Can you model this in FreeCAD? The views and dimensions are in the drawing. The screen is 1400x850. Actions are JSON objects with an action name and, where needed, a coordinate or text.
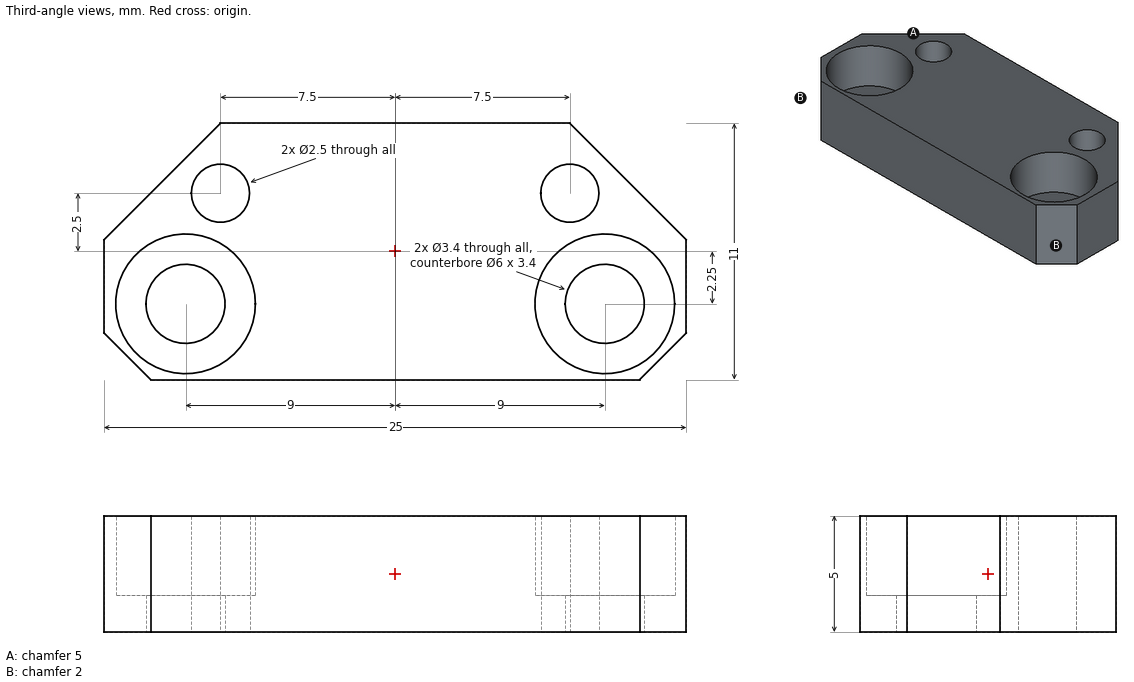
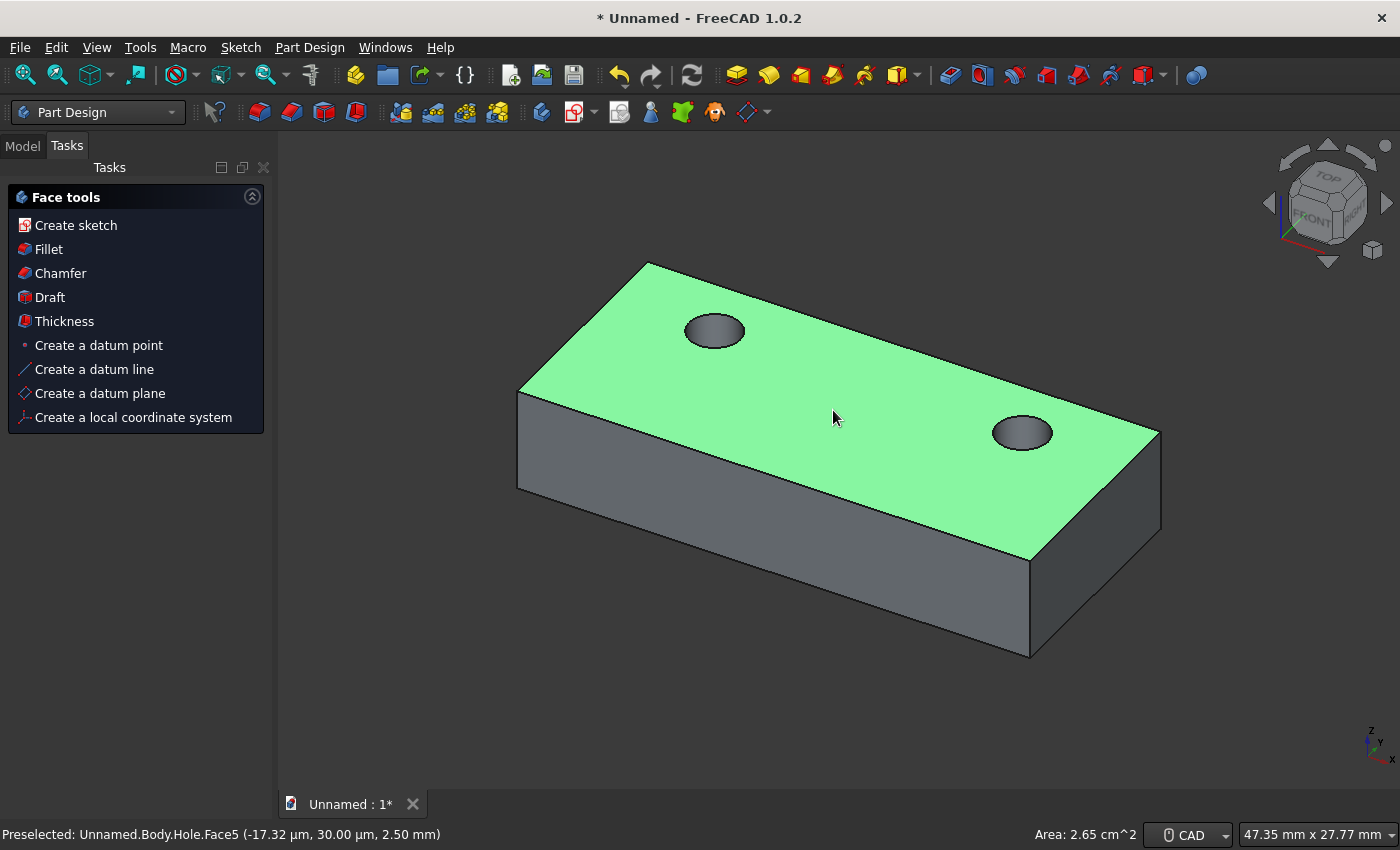
{"action": "left_click", "coordinate": [574, 112]}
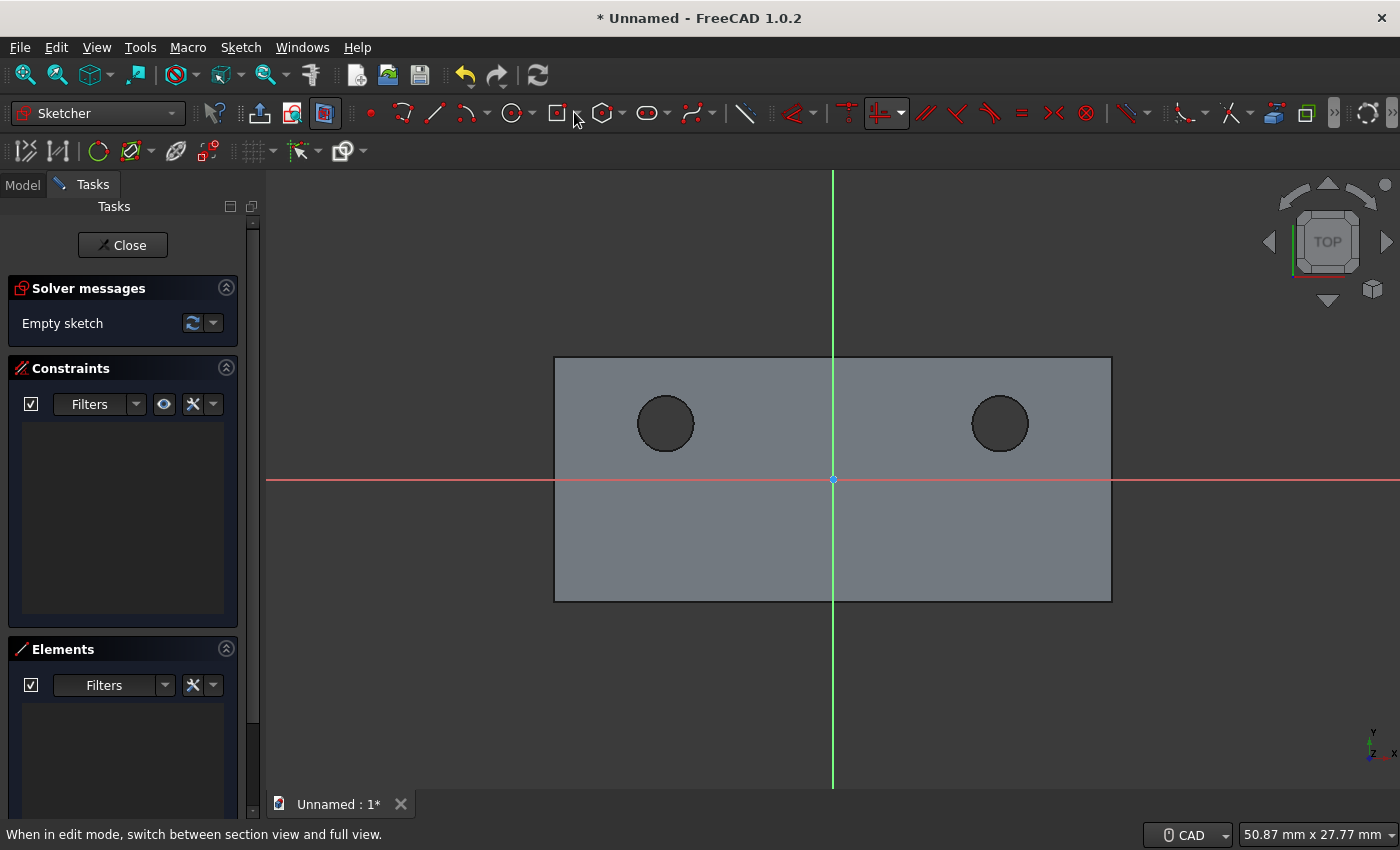
{"action": "scroll", "coordinate": [972, 613], "scroll_direction": "up", "scroll_amount": 2}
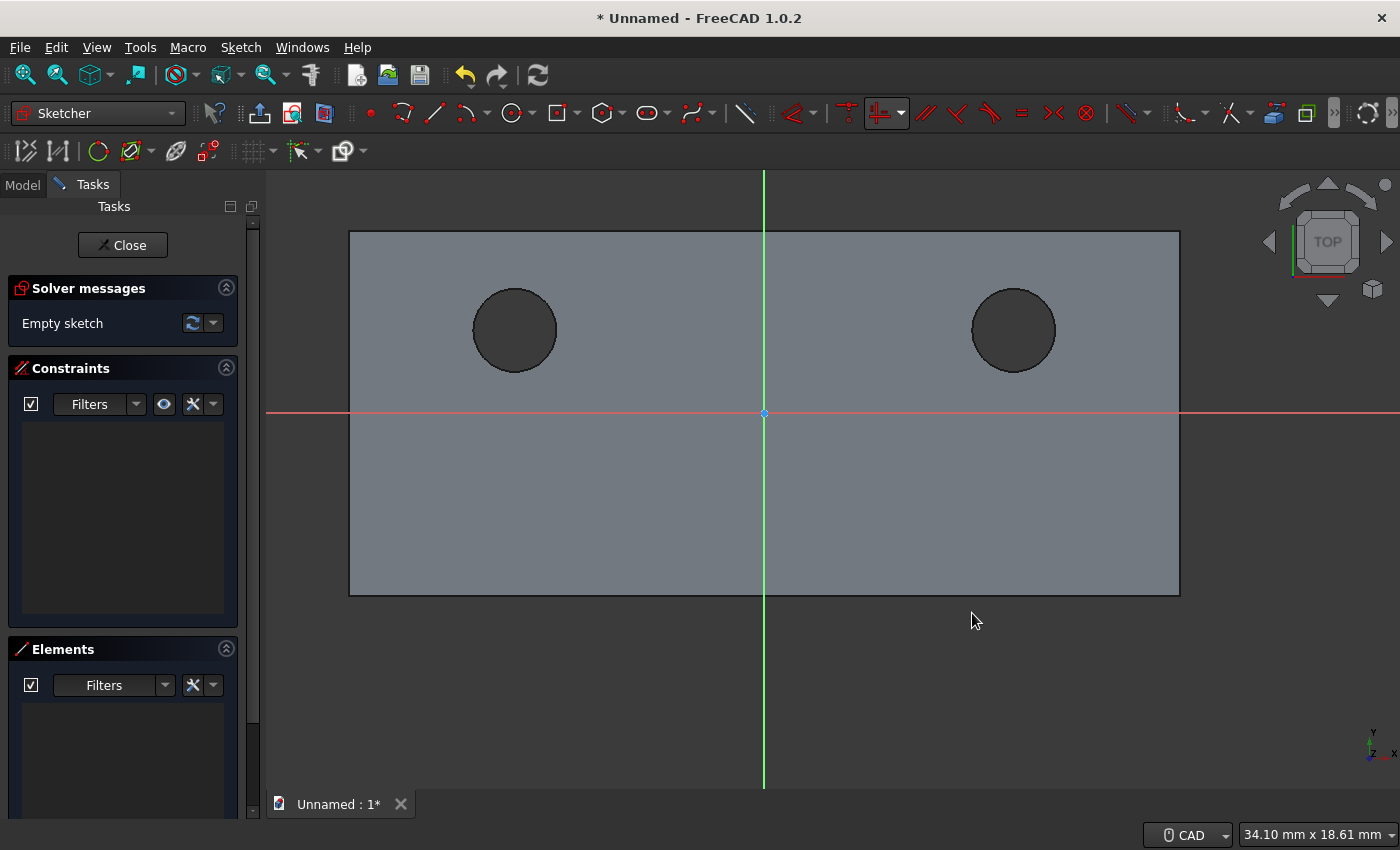
{"action": "left_click", "coordinate": [512, 114]}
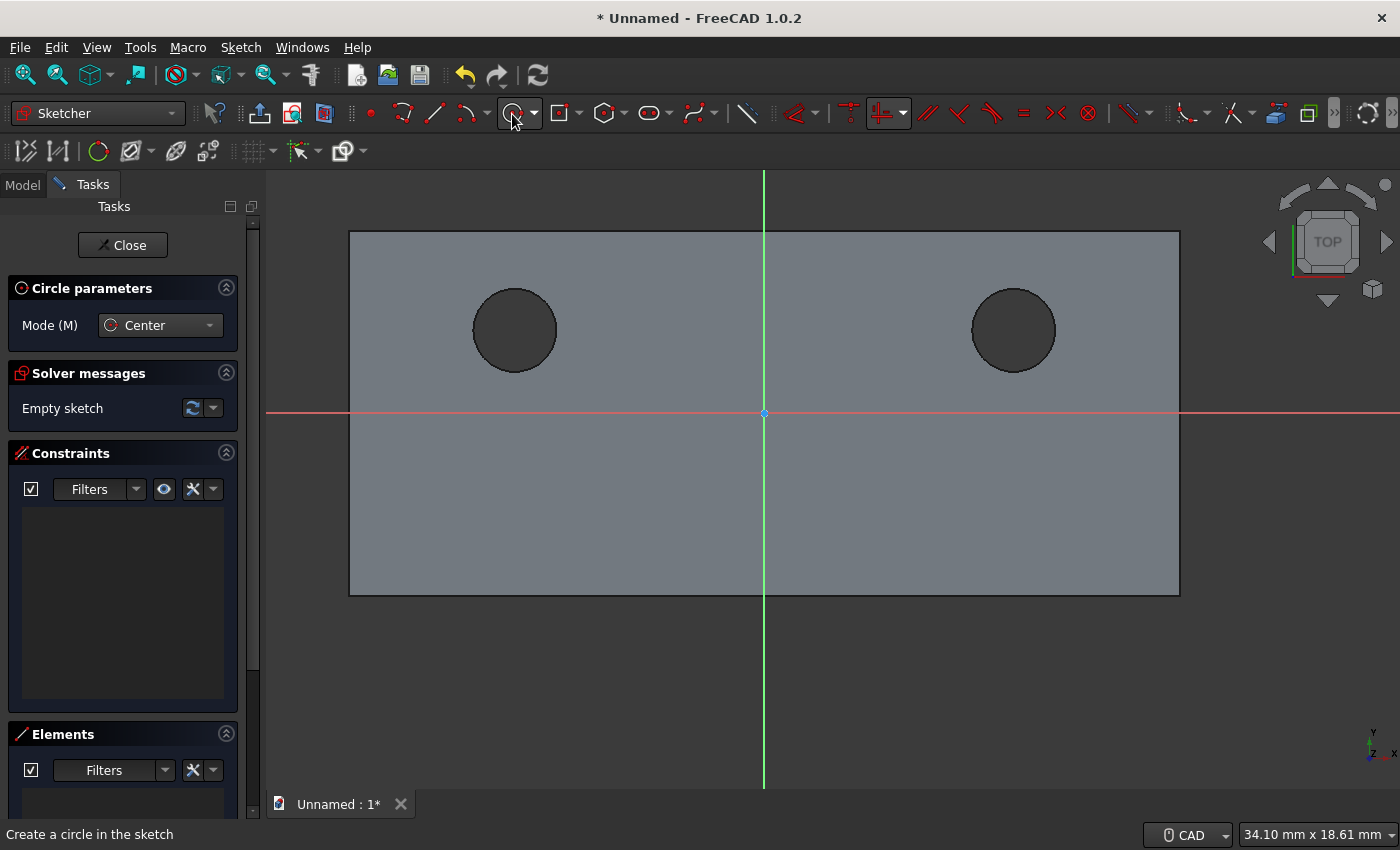
{"action": "left_click", "coordinate": [1064, 488]}
{"action": "left_click", "coordinate": [1104, 448]}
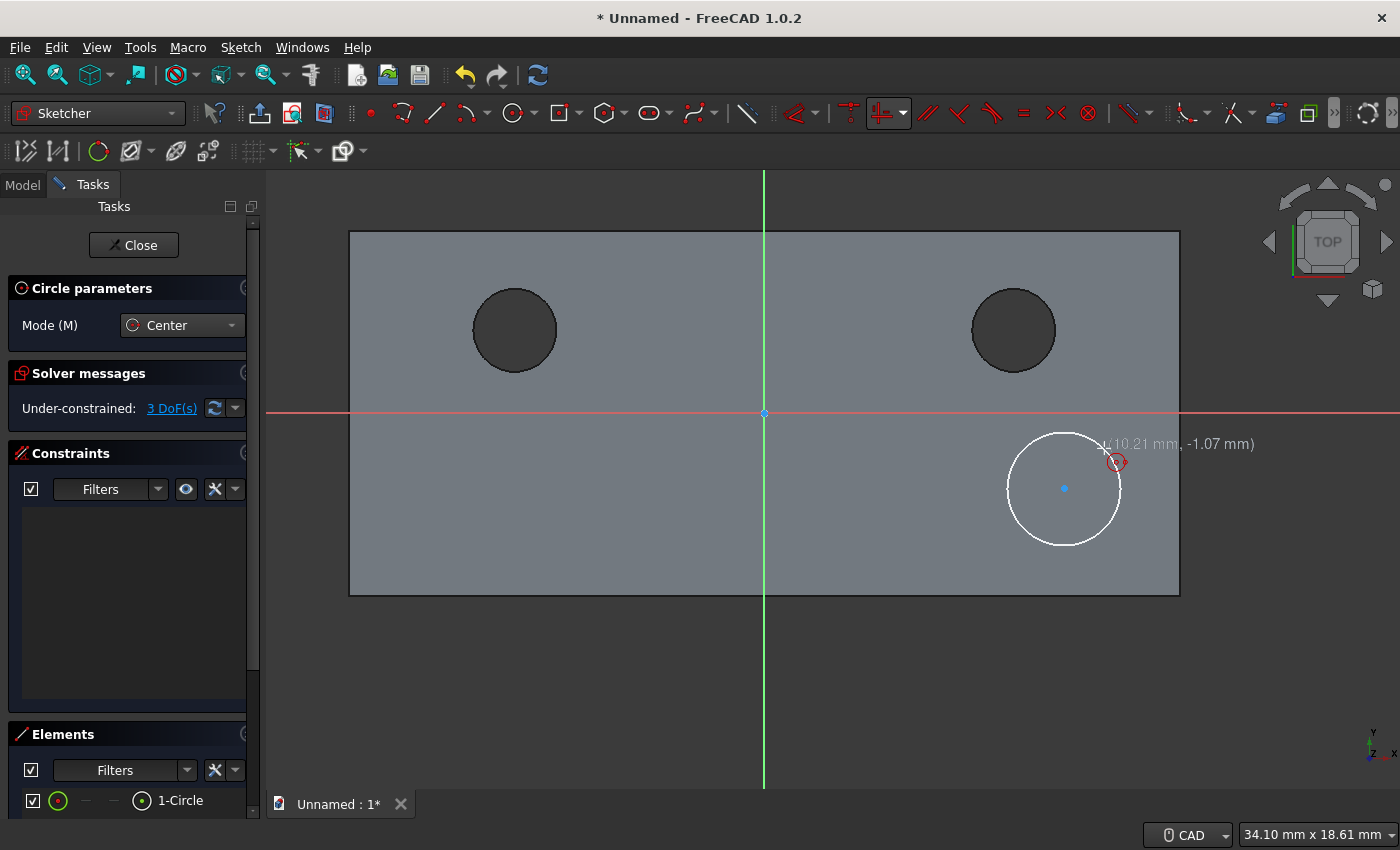
{"action": "left_click", "coordinate": [465, 488]}
{"action": "left_click", "coordinate": [505, 448]}
{"action": "key", "text": "Escape"}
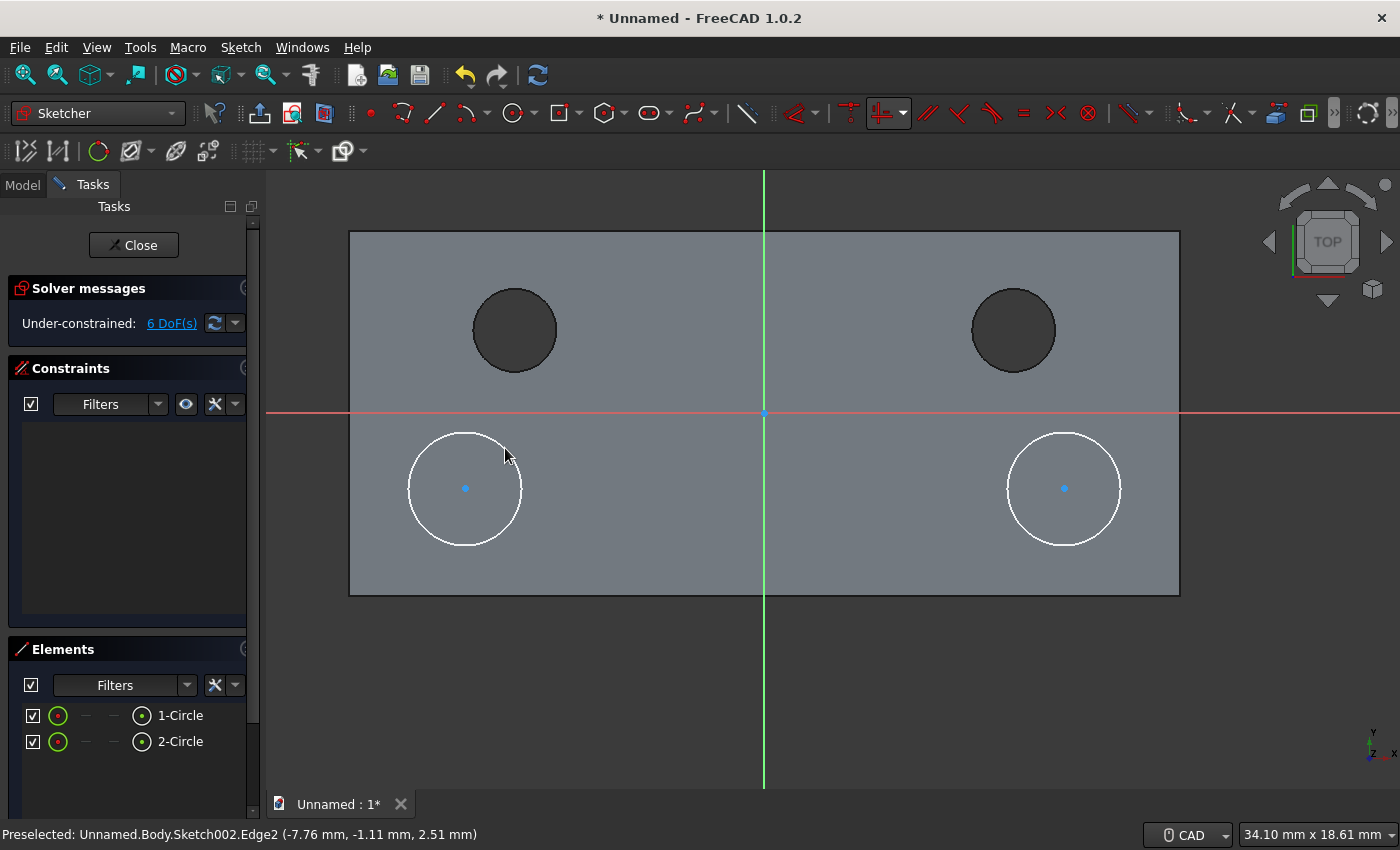
{"action": "left_click", "coordinate": [1104, 449]}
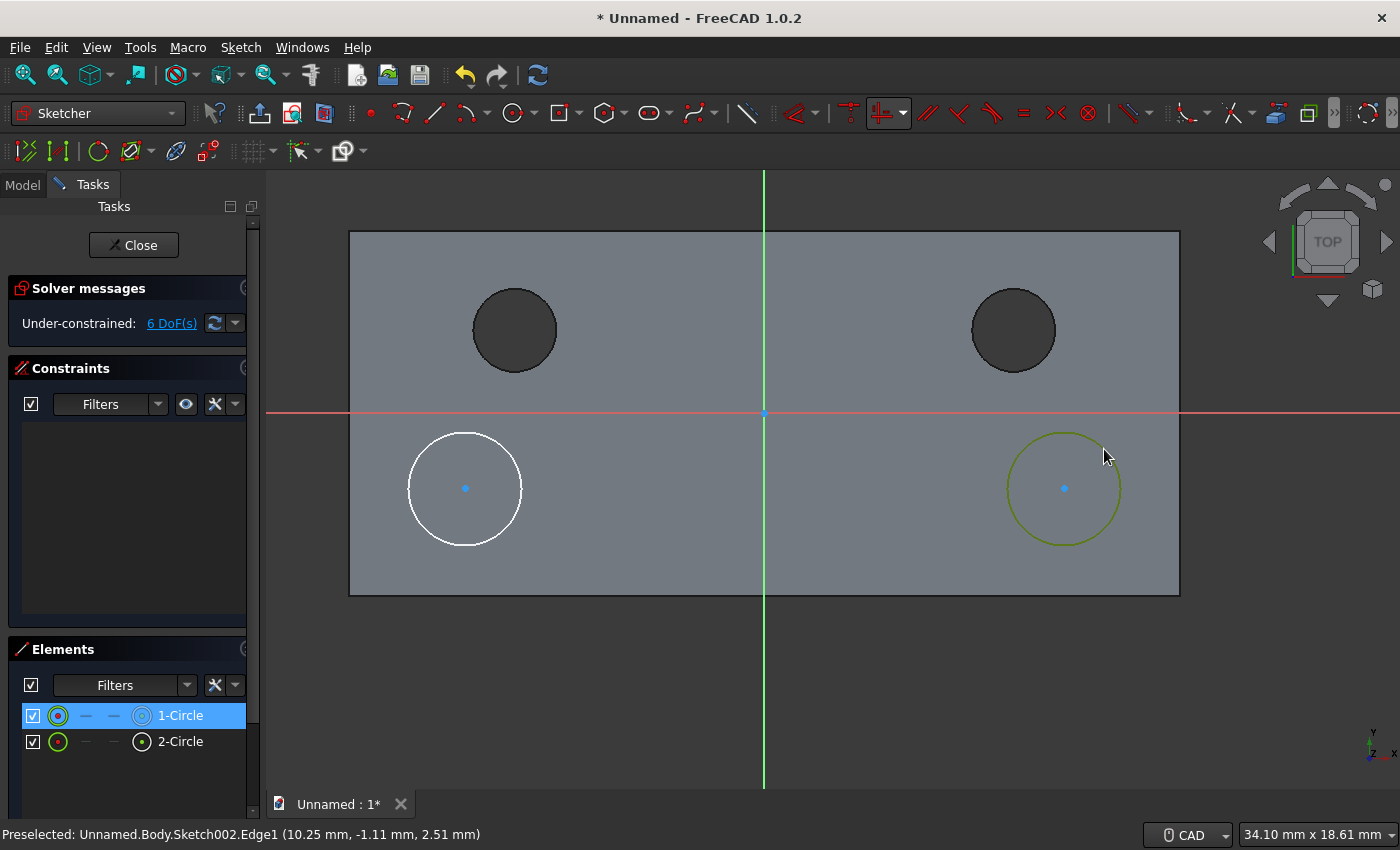
{"action": "left_click", "coordinate": [505, 449]}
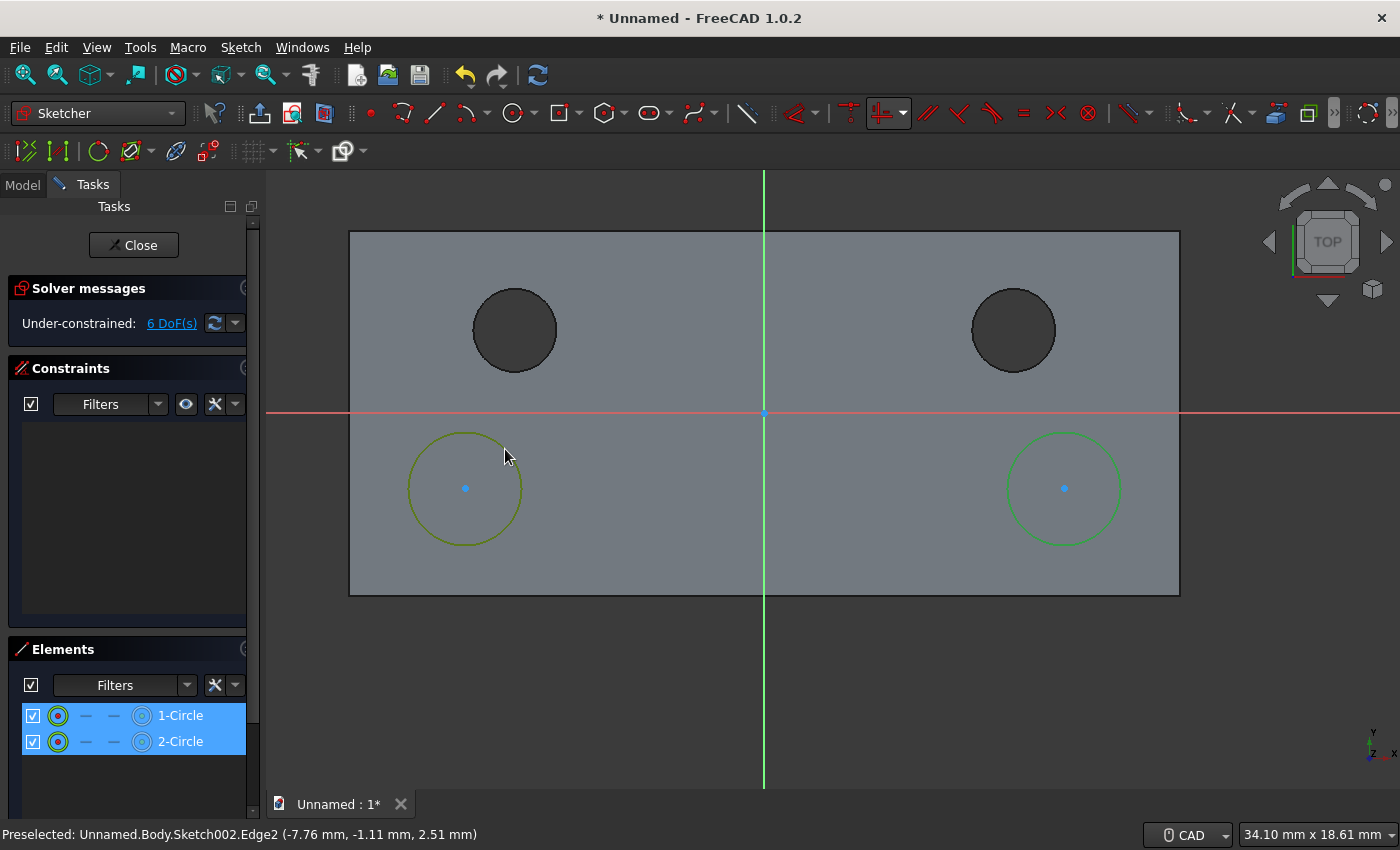
{"action": "left_click", "coordinate": [1024, 114]}